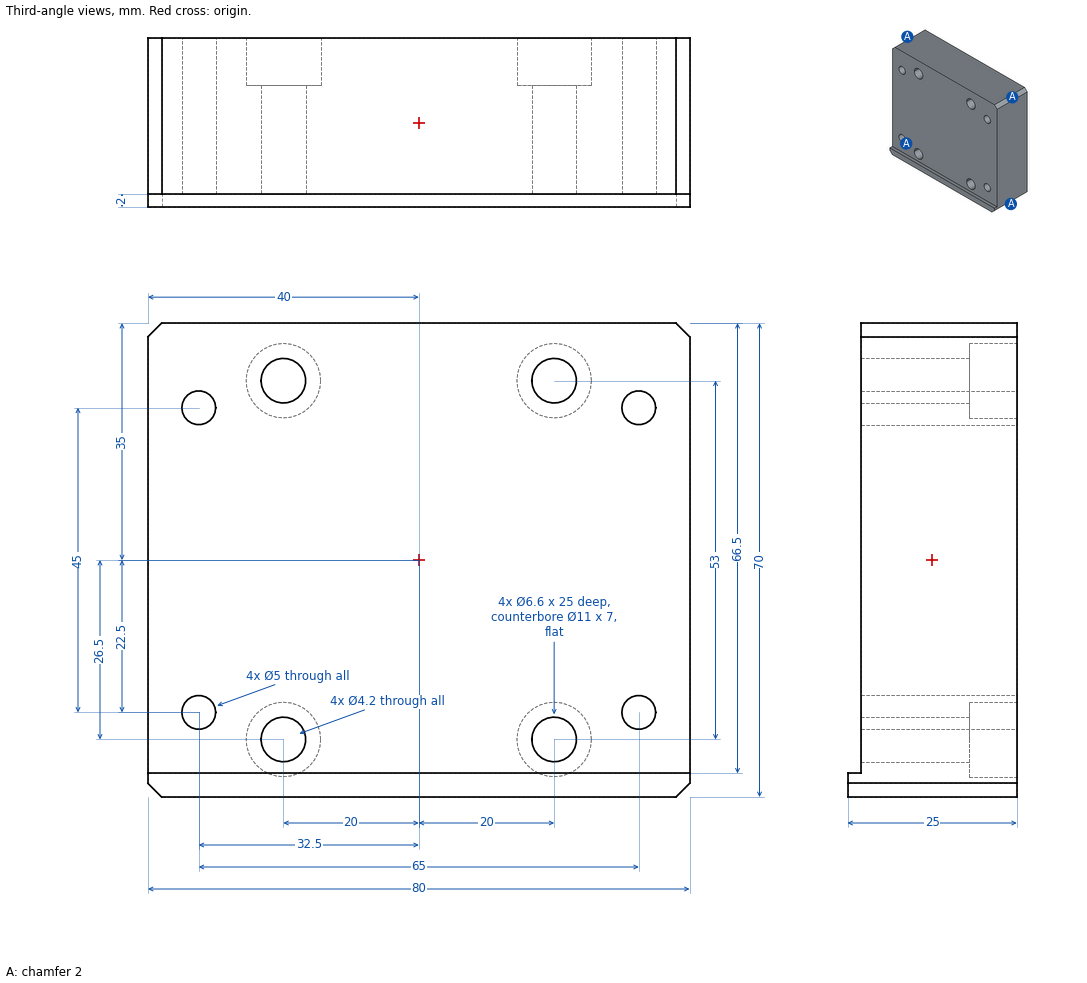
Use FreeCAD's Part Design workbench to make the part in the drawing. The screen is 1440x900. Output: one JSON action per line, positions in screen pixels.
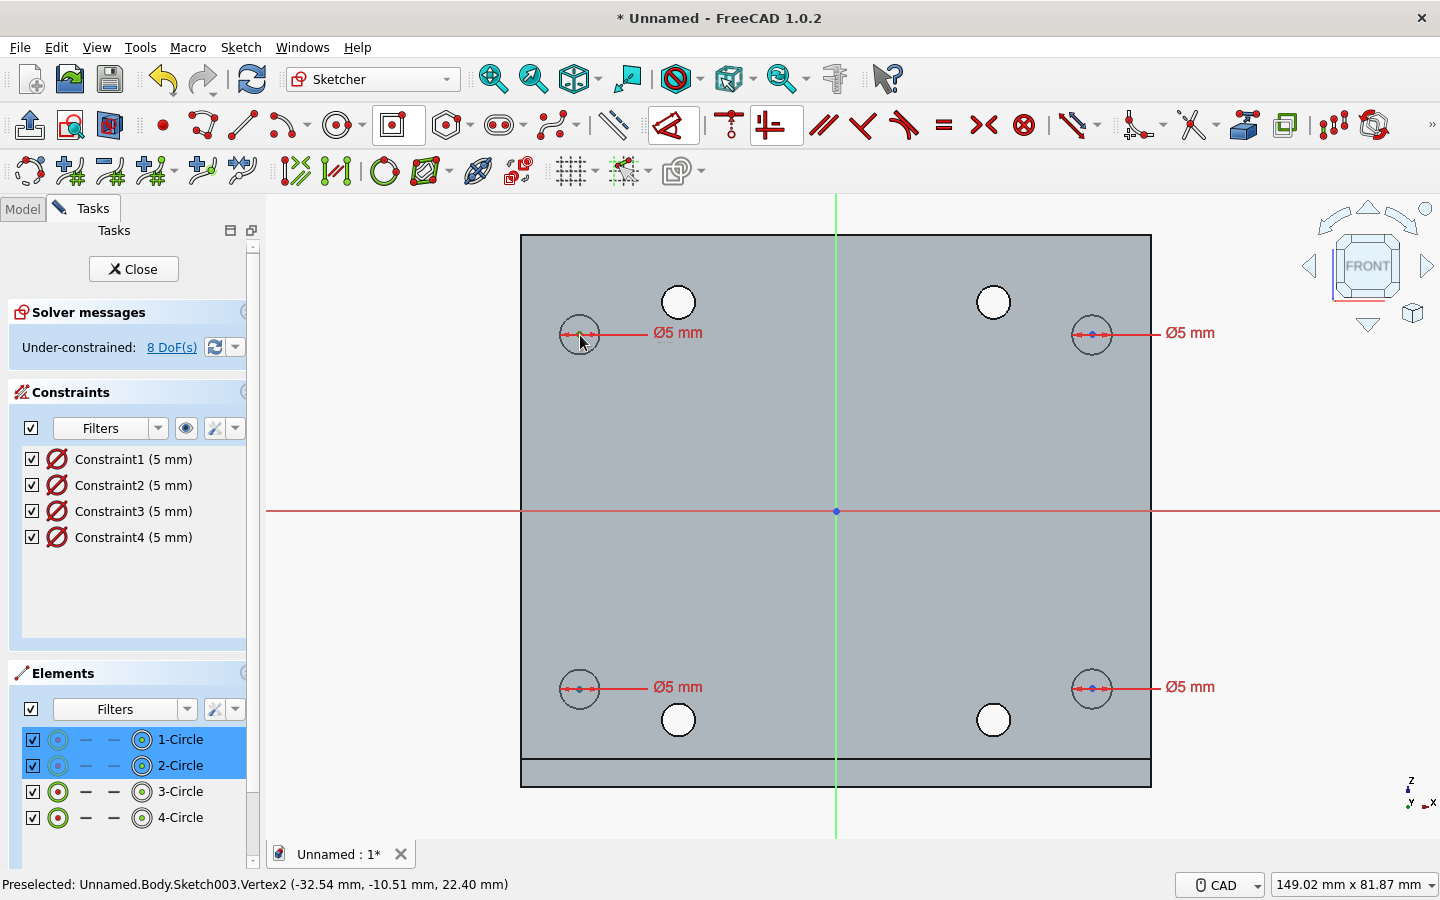
{"action": "left_click", "coordinate": [798, 126]}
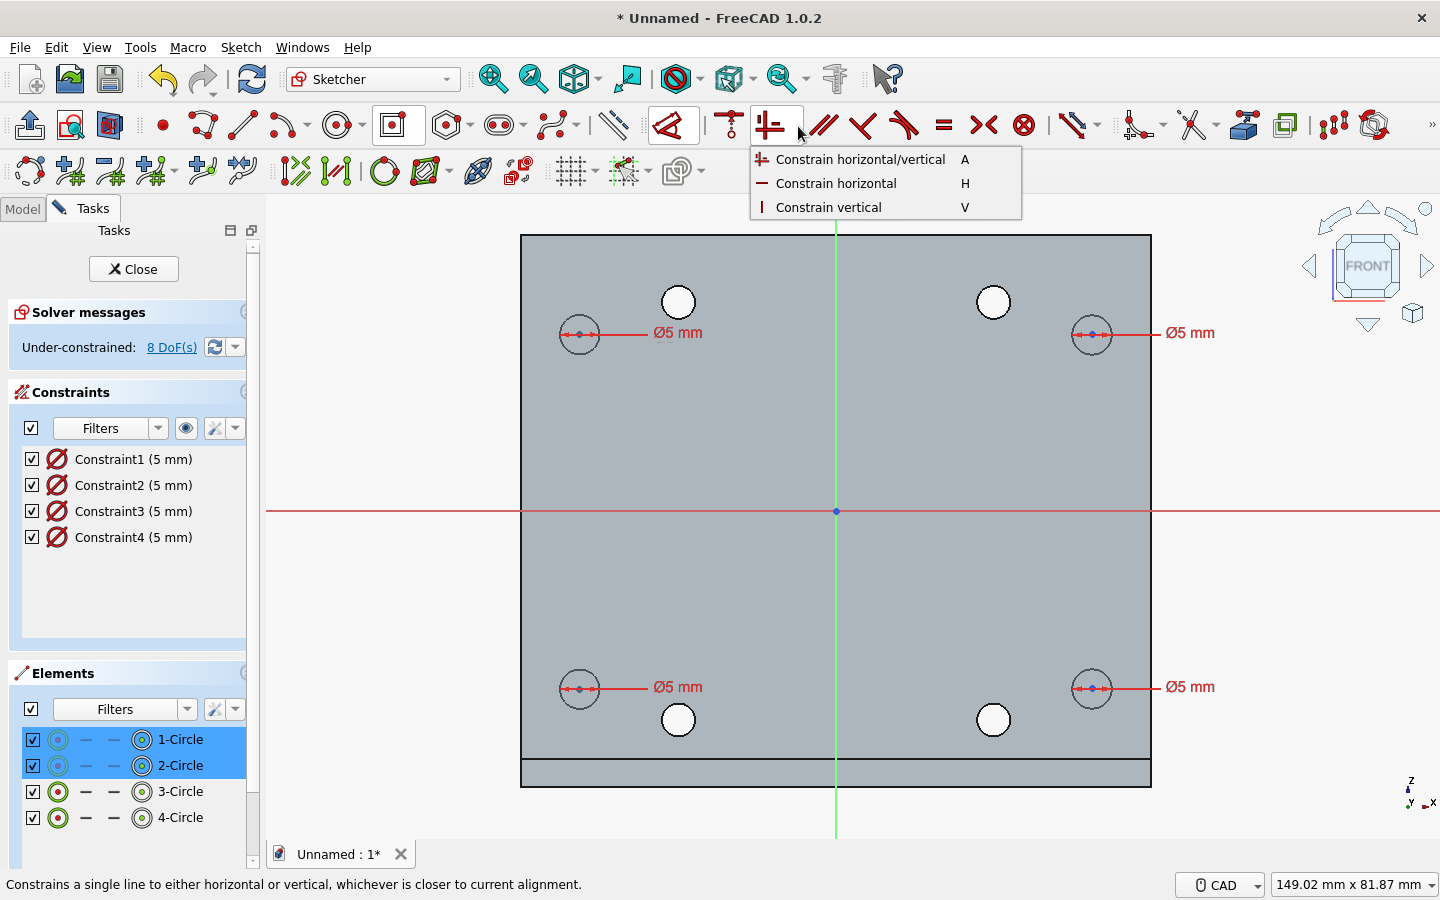
{"action": "left_click", "coordinate": [886, 207]}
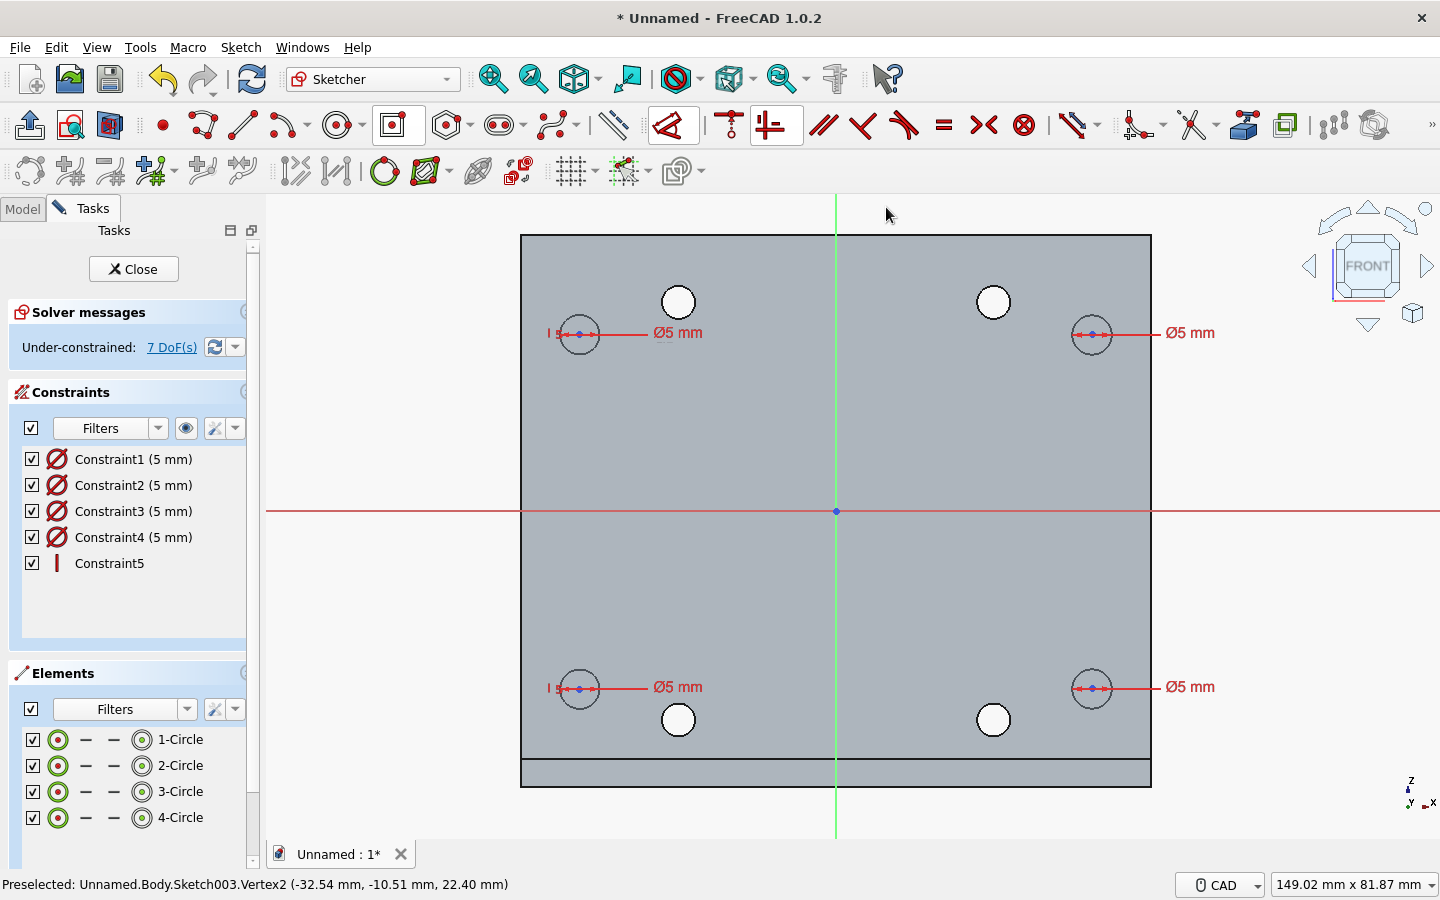
{"action": "left_click", "coordinate": [580, 689]}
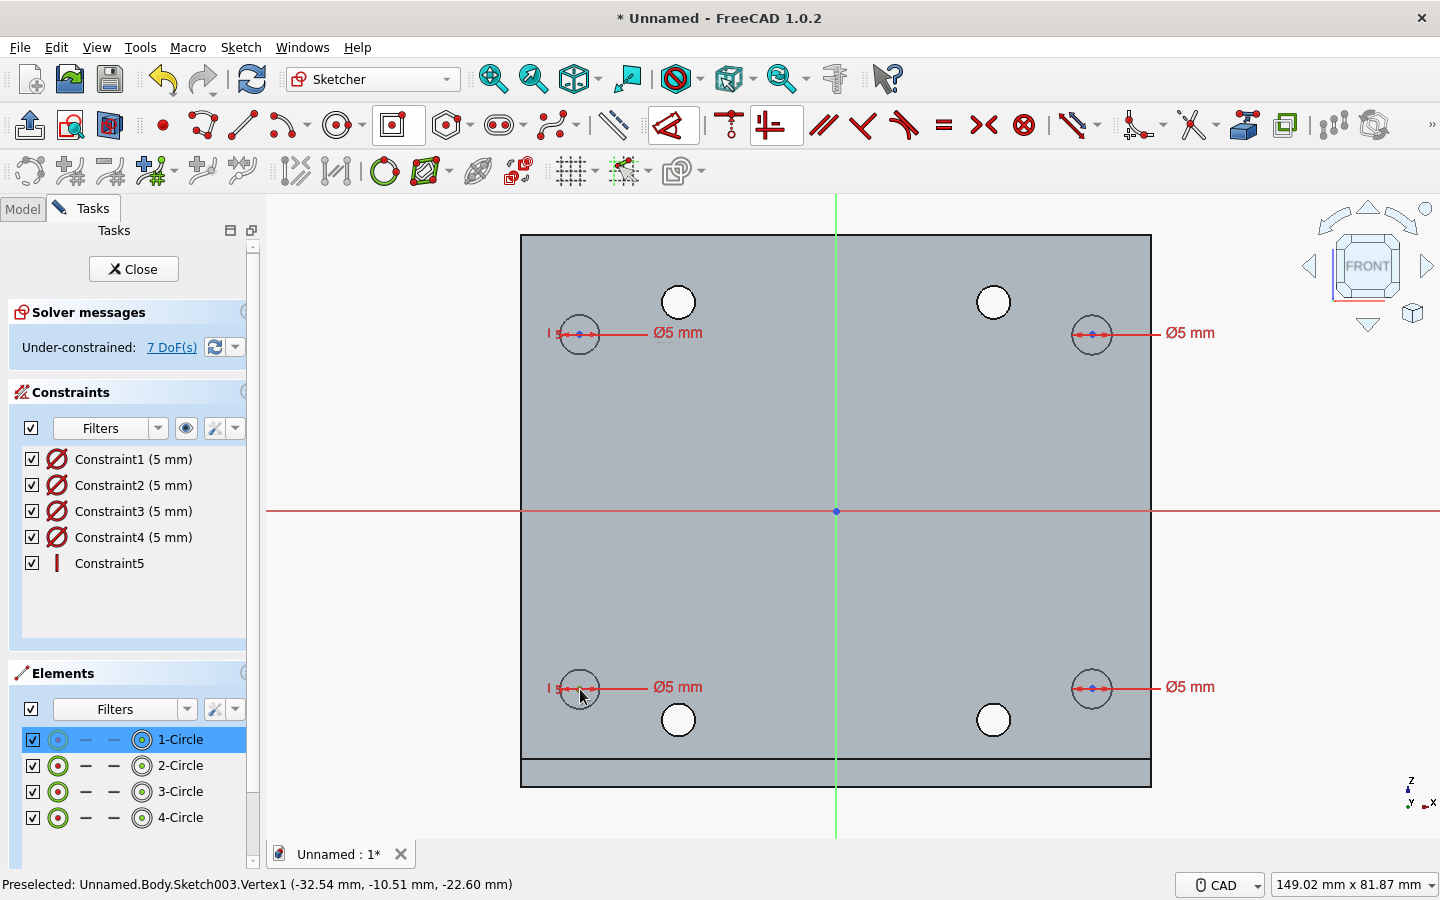
{"action": "left_click", "coordinate": [1092, 689]}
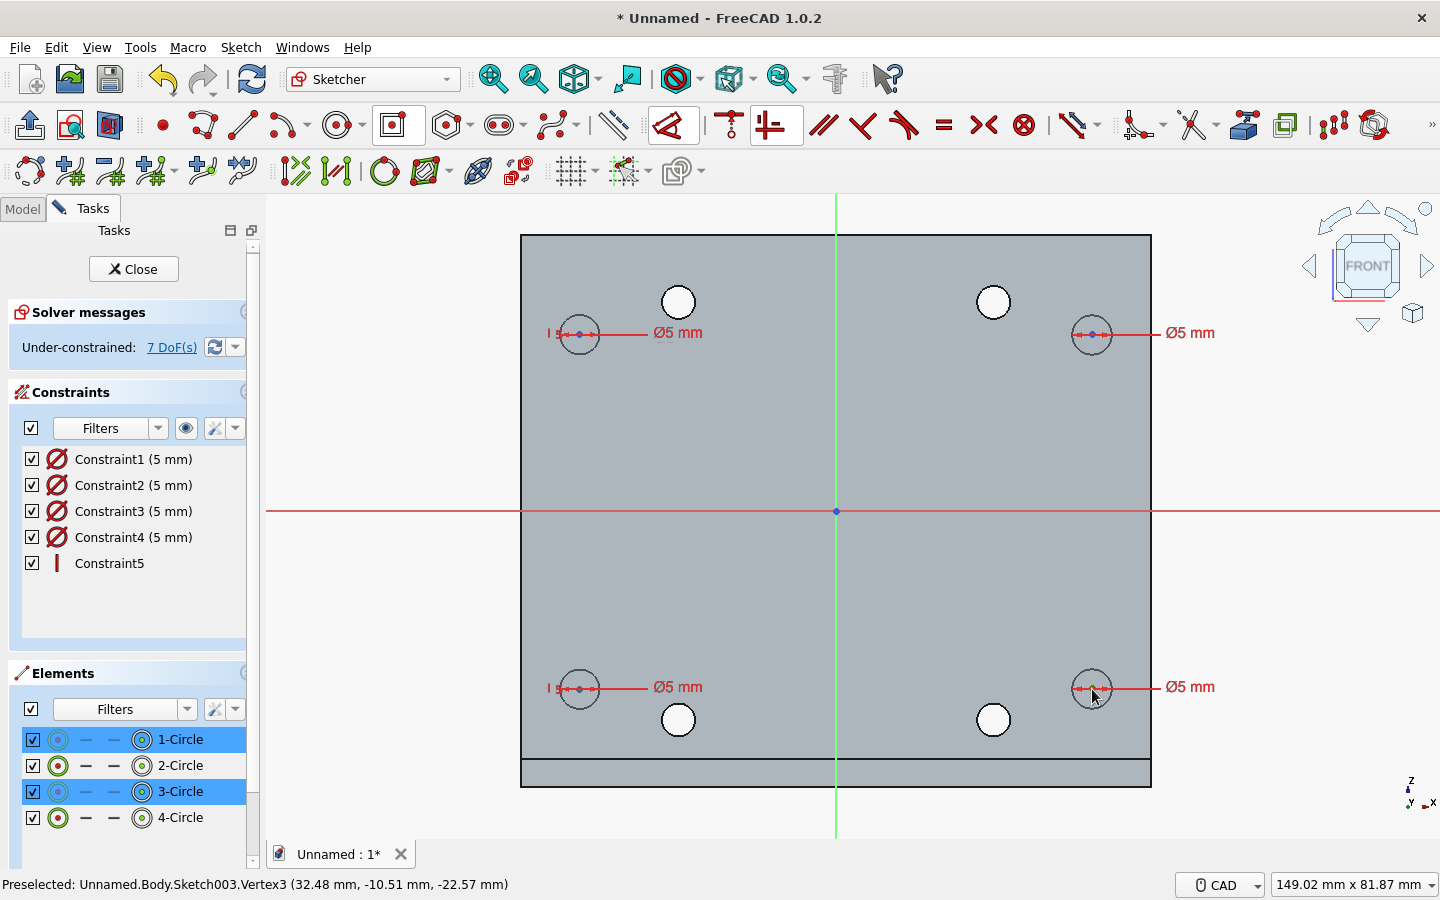
{"action": "left_click", "coordinate": [798, 126]}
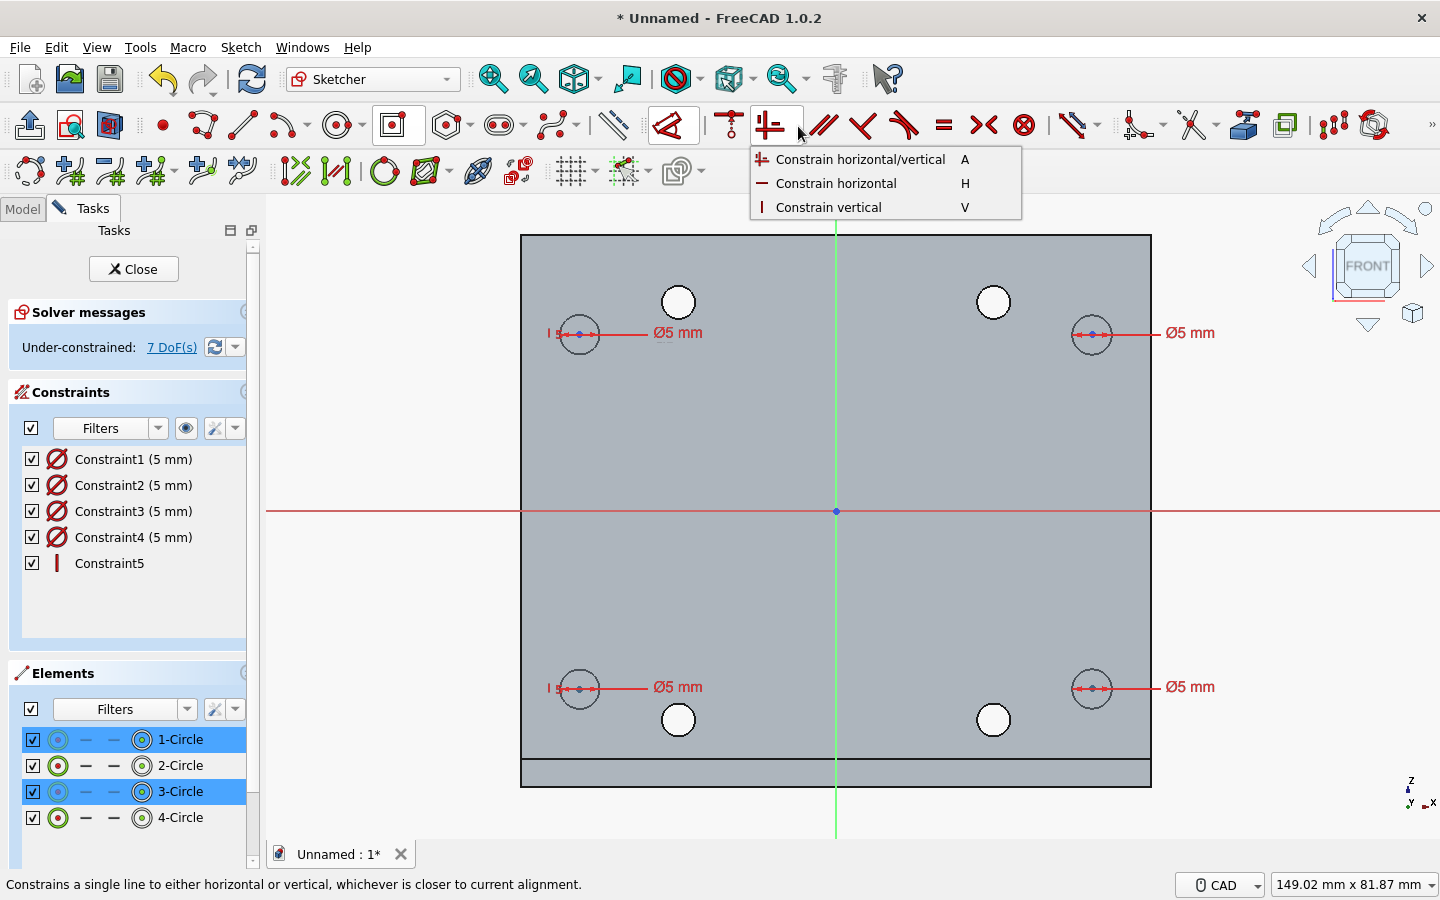
{"action": "left_click", "coordinate": [886, 183]}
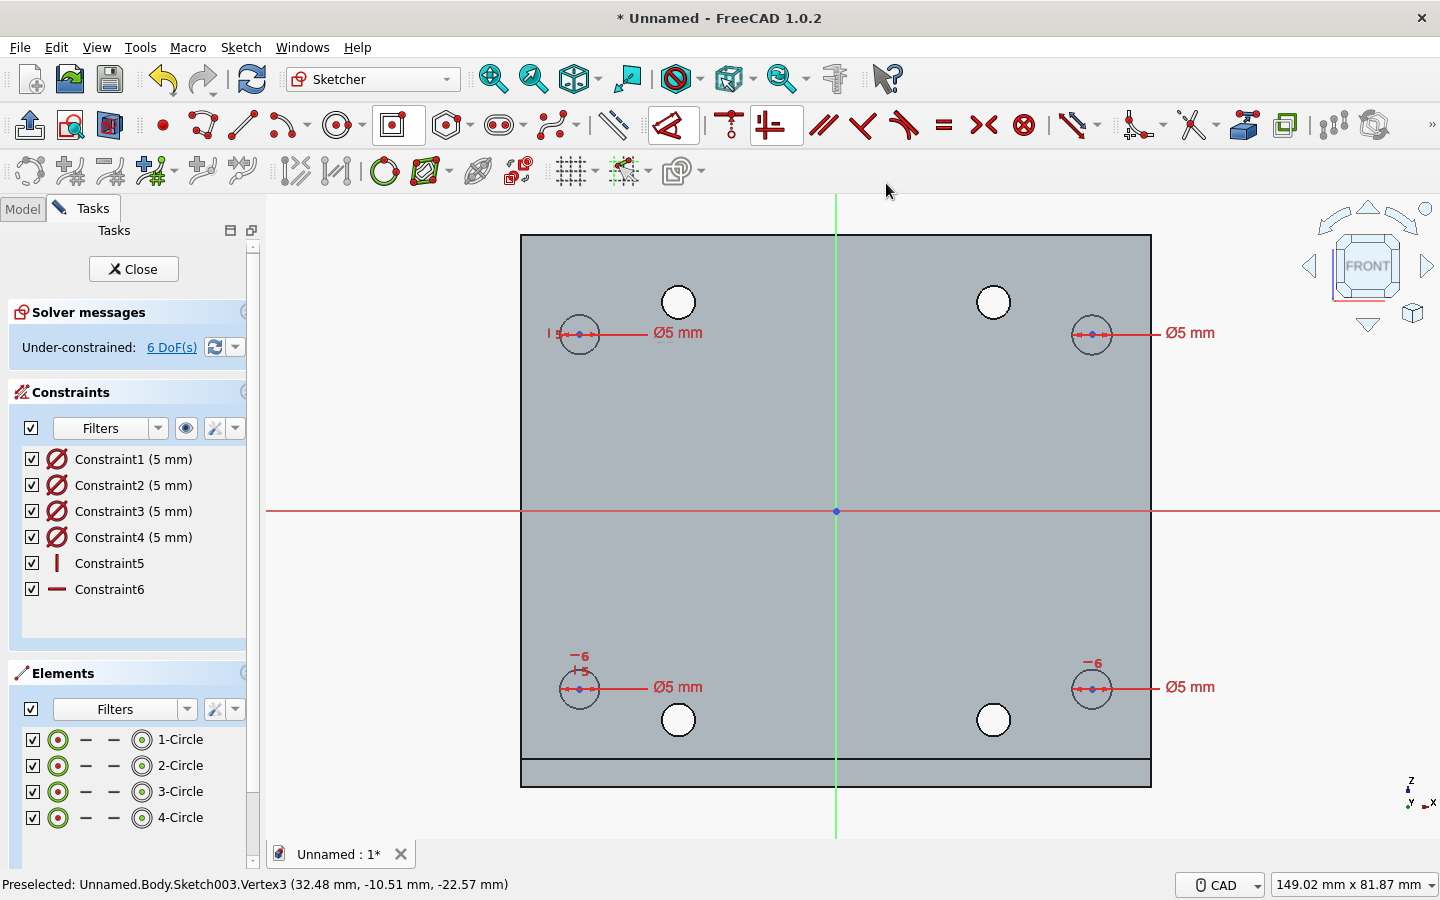
{"action": "left_click", "coordinate": [1092, 689]}